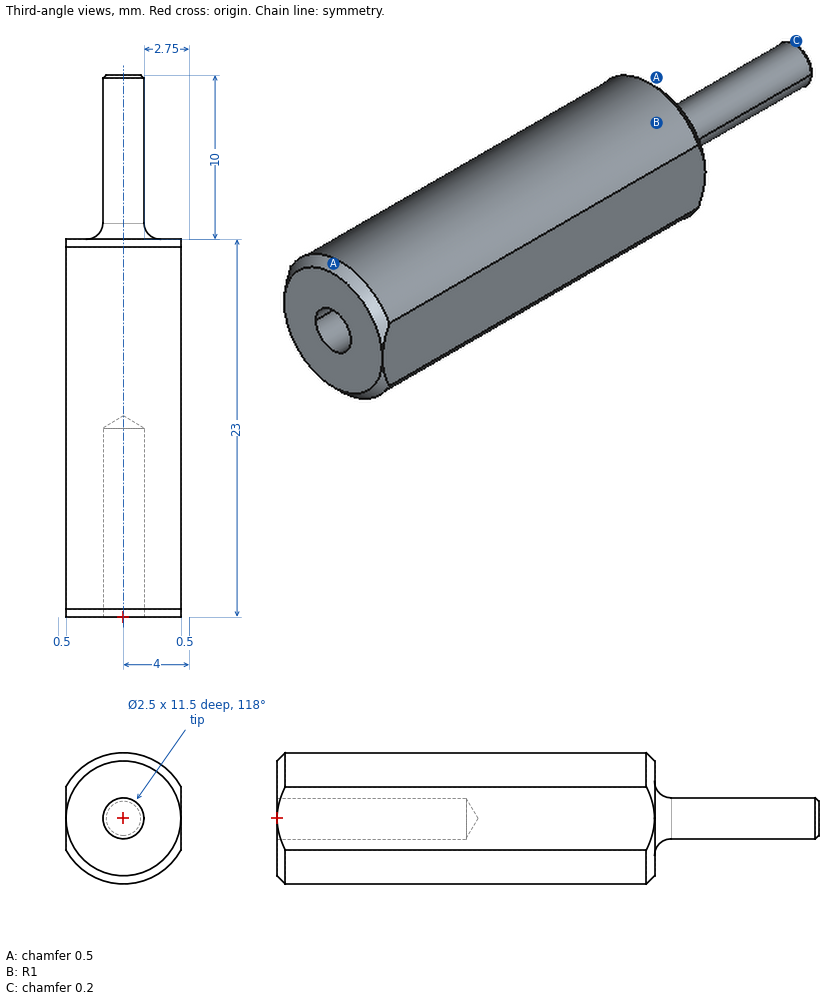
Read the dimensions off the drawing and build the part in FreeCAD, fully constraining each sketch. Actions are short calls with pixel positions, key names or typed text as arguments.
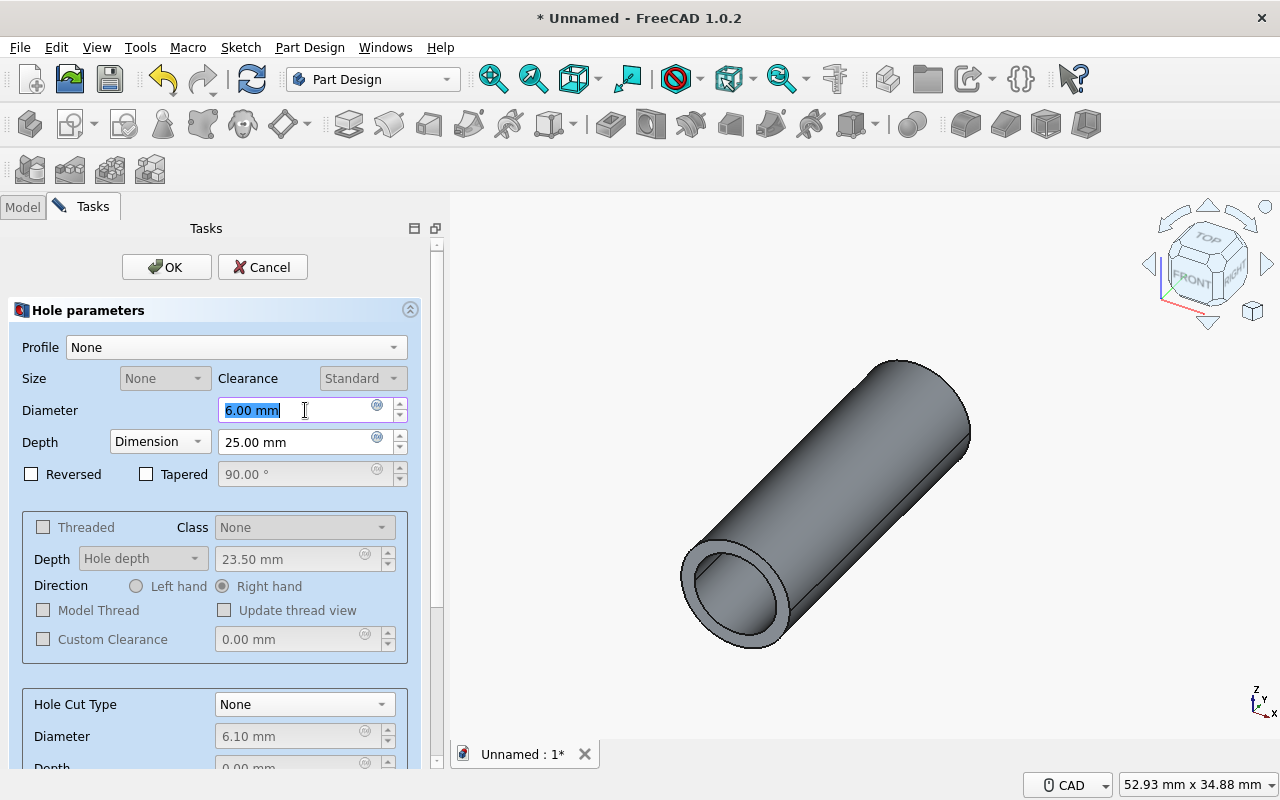
text(2.5)
key(Tab)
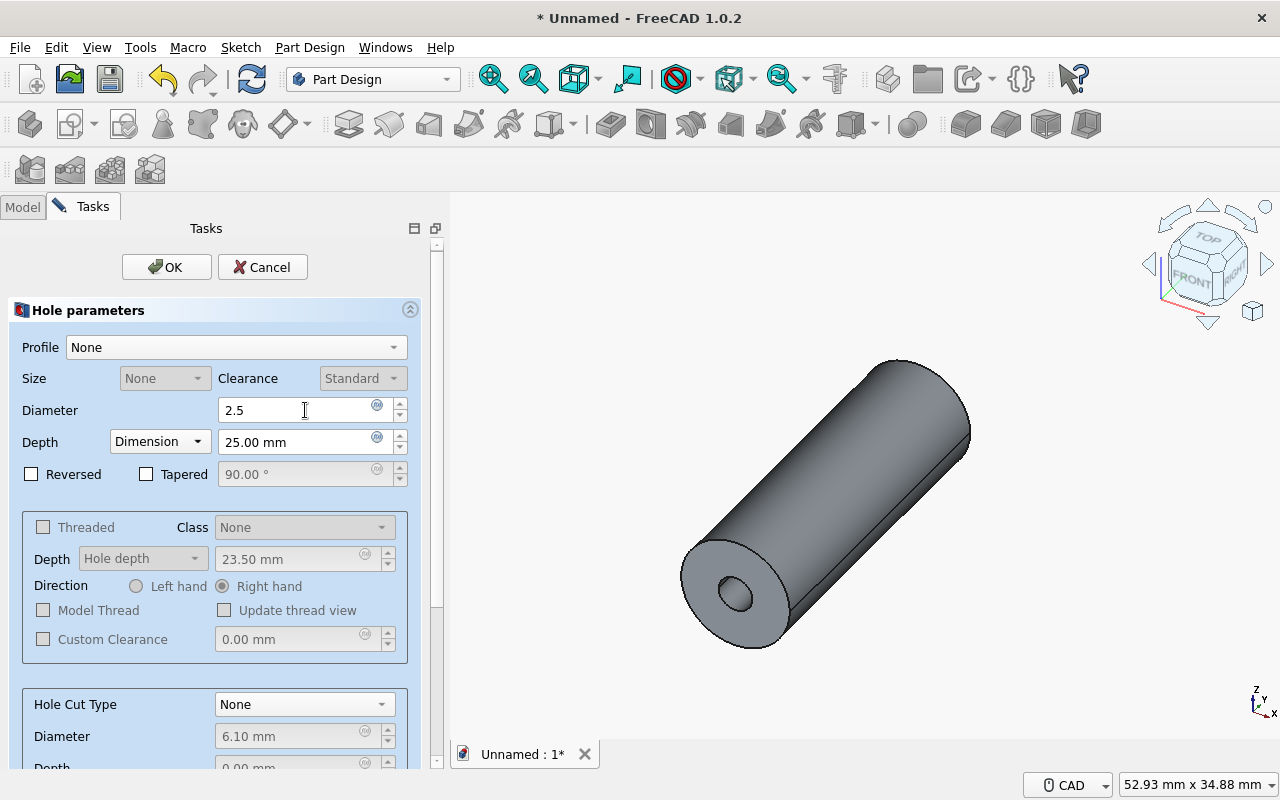
triple_click(305, 442)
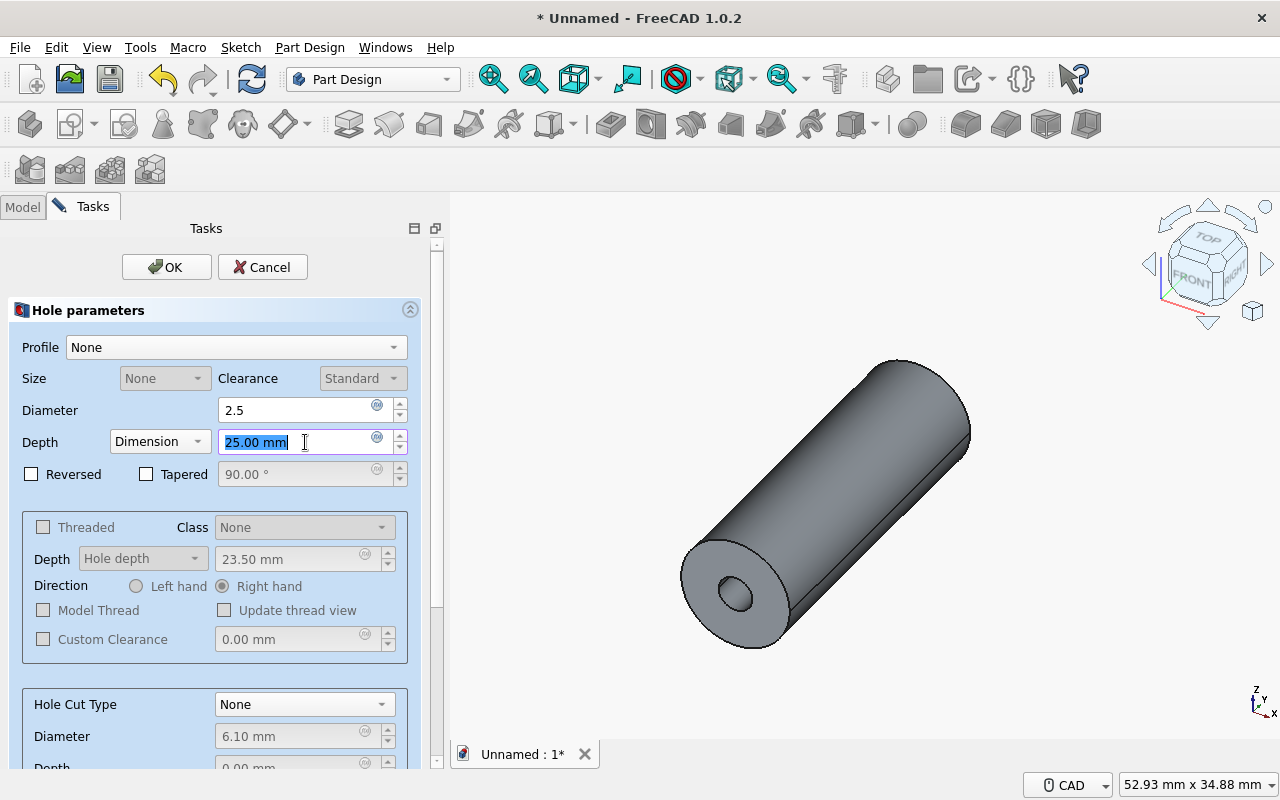
text(11.5)
key(Tab)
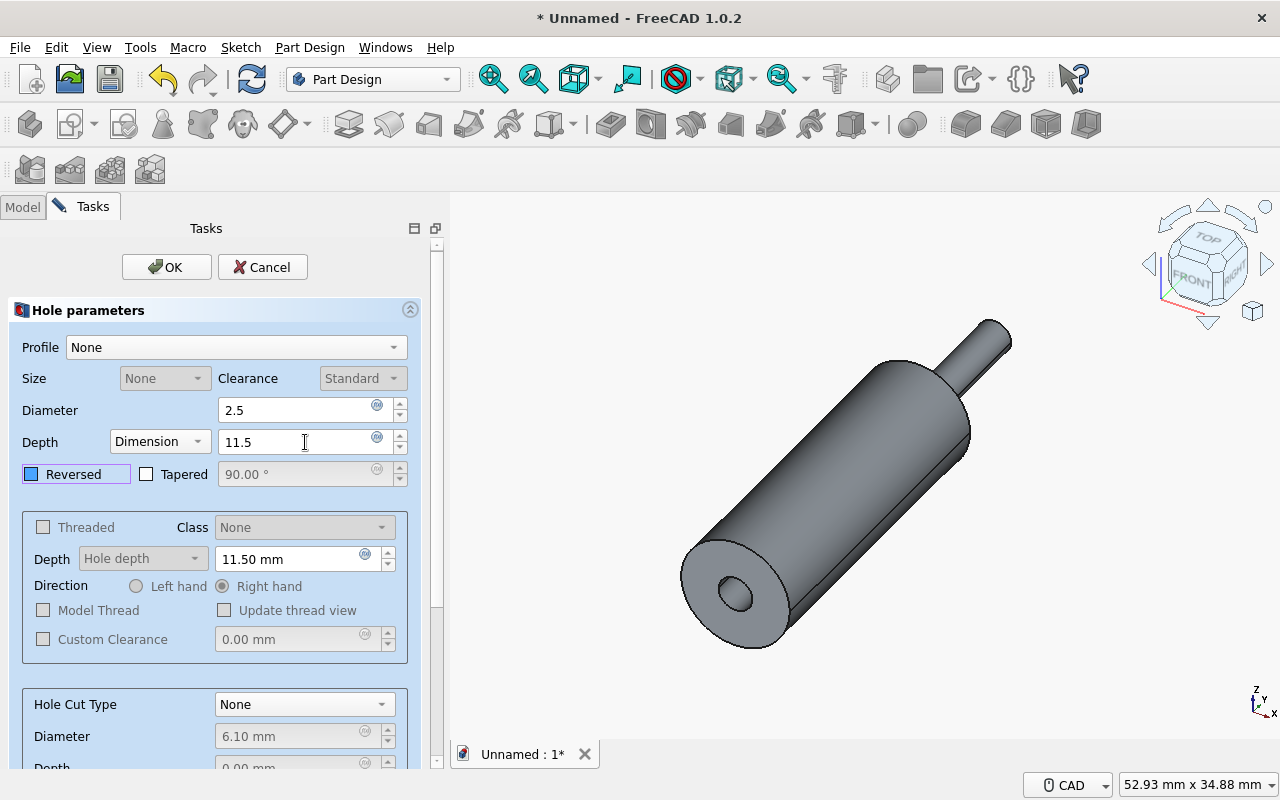
click(167, 267)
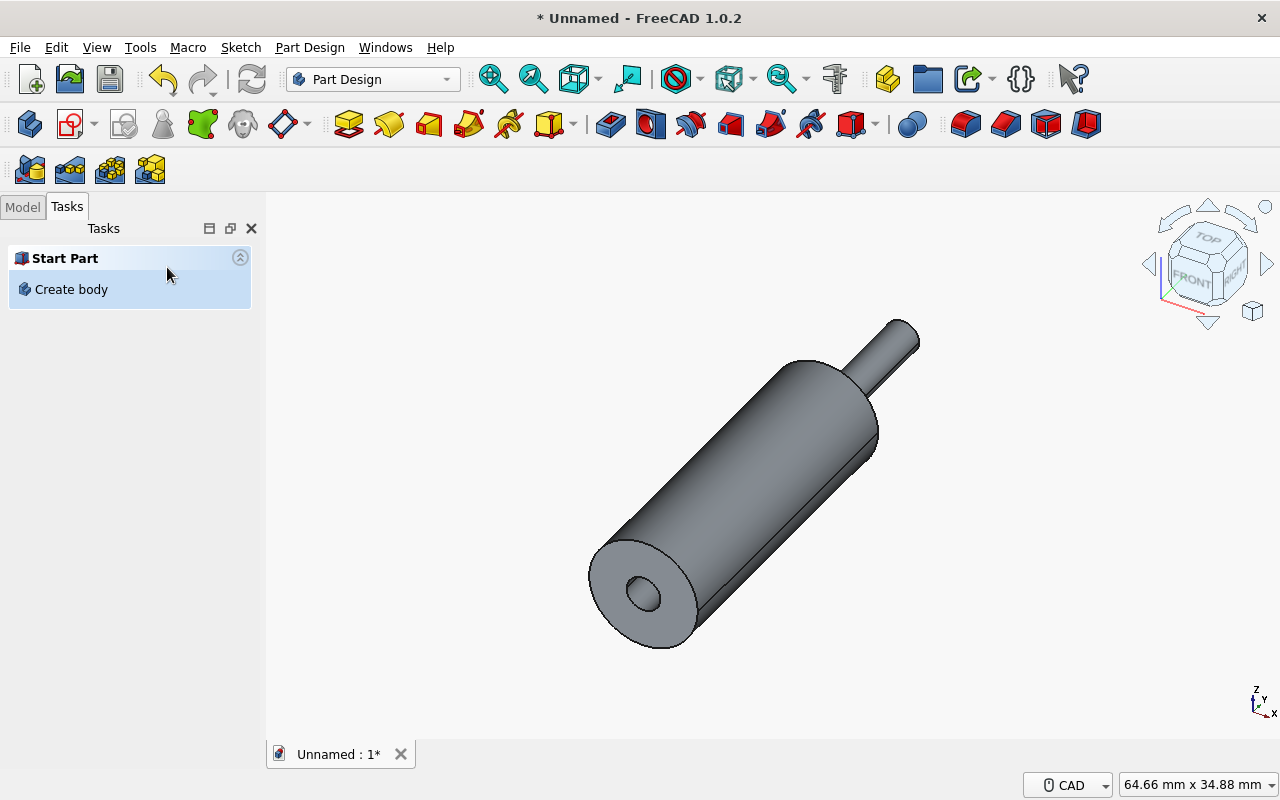
click(600, 548)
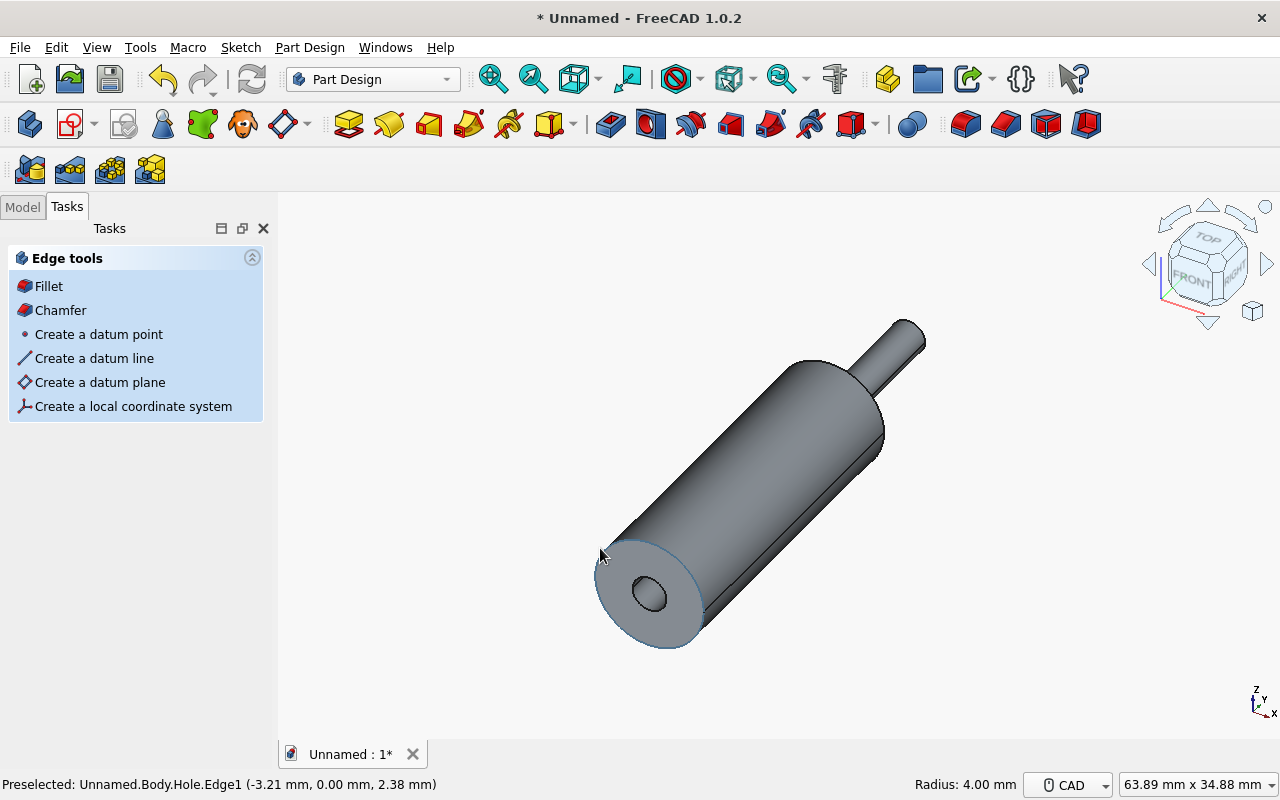
key(0)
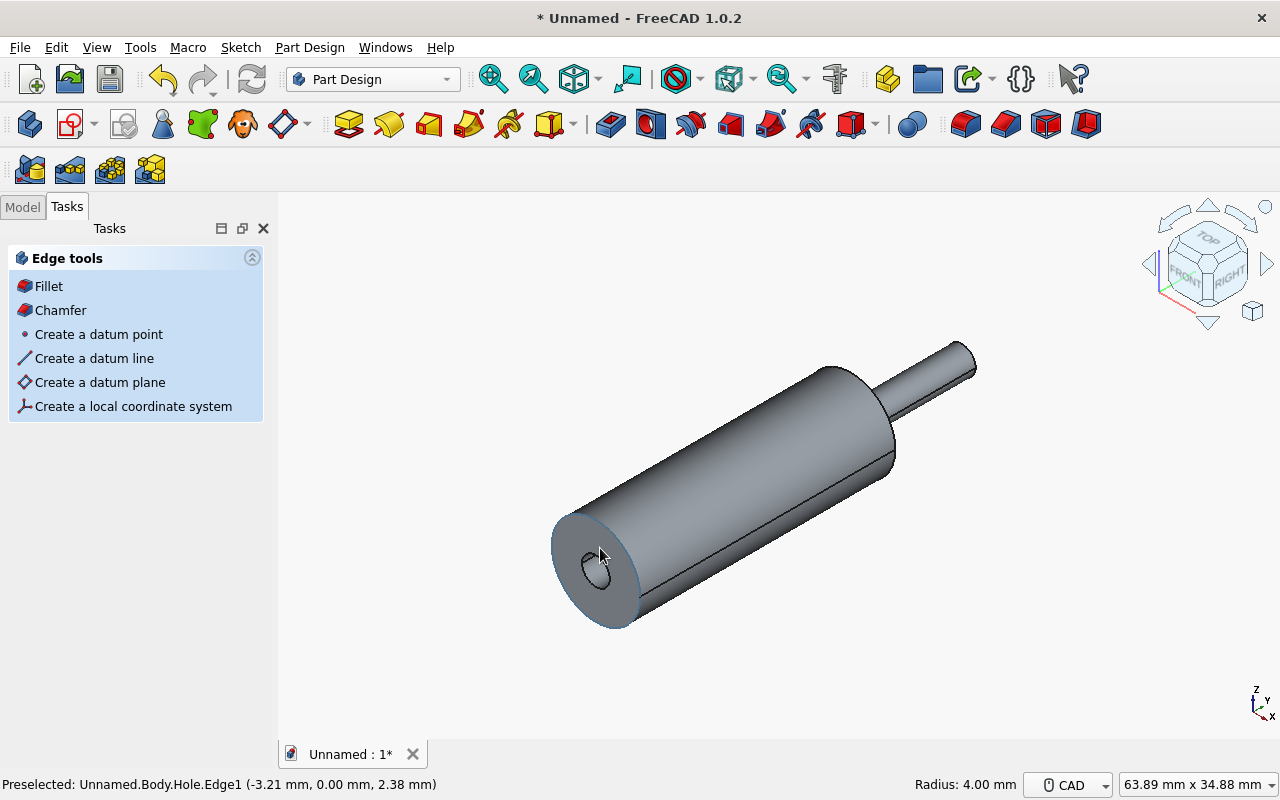
key(2)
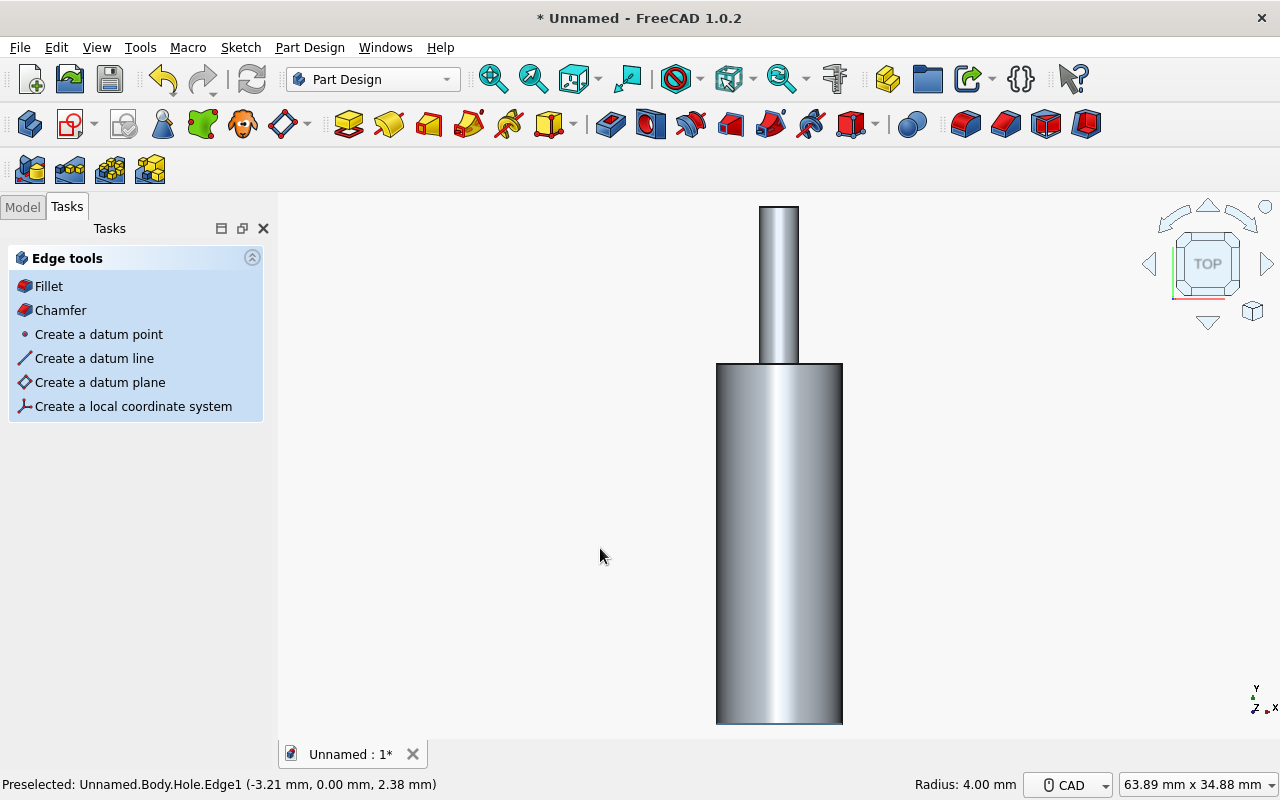
click(728, 363, ctrl)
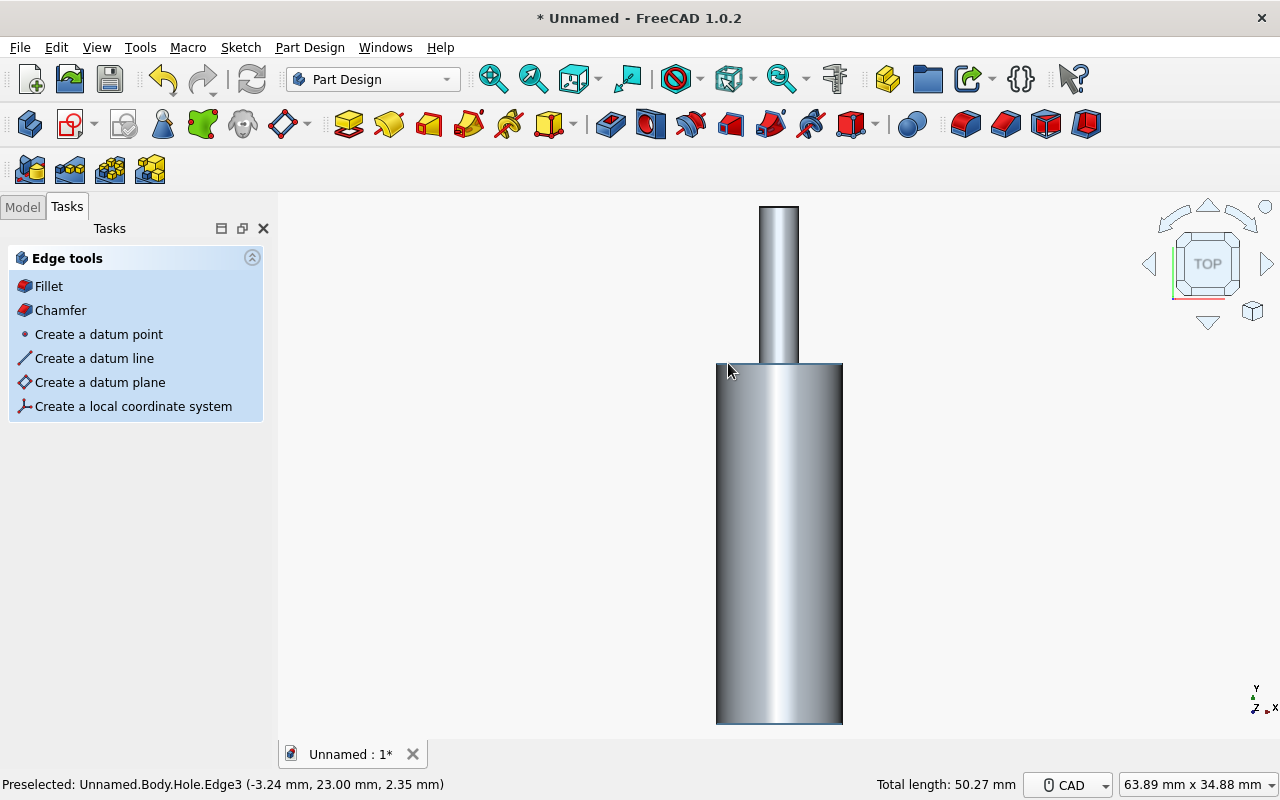
click(1006, 124)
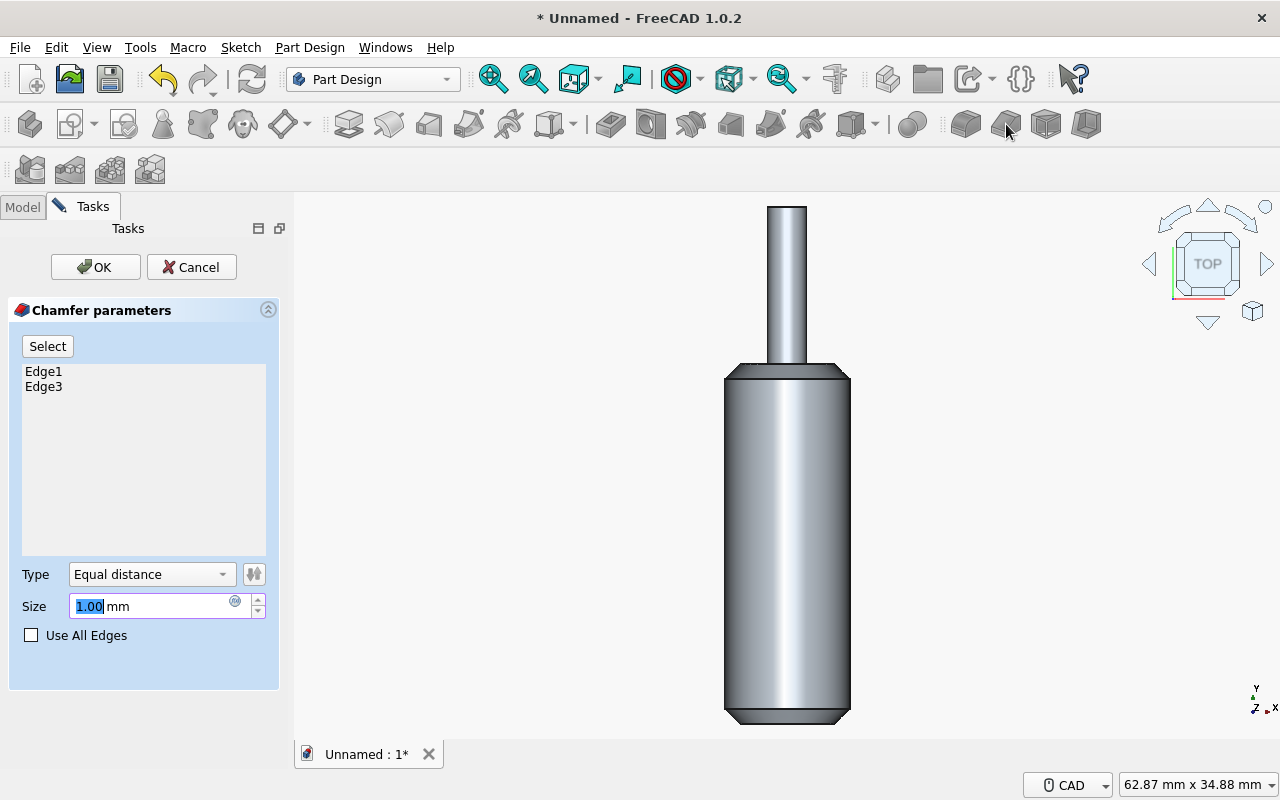
text(0.5)
key(Tab)